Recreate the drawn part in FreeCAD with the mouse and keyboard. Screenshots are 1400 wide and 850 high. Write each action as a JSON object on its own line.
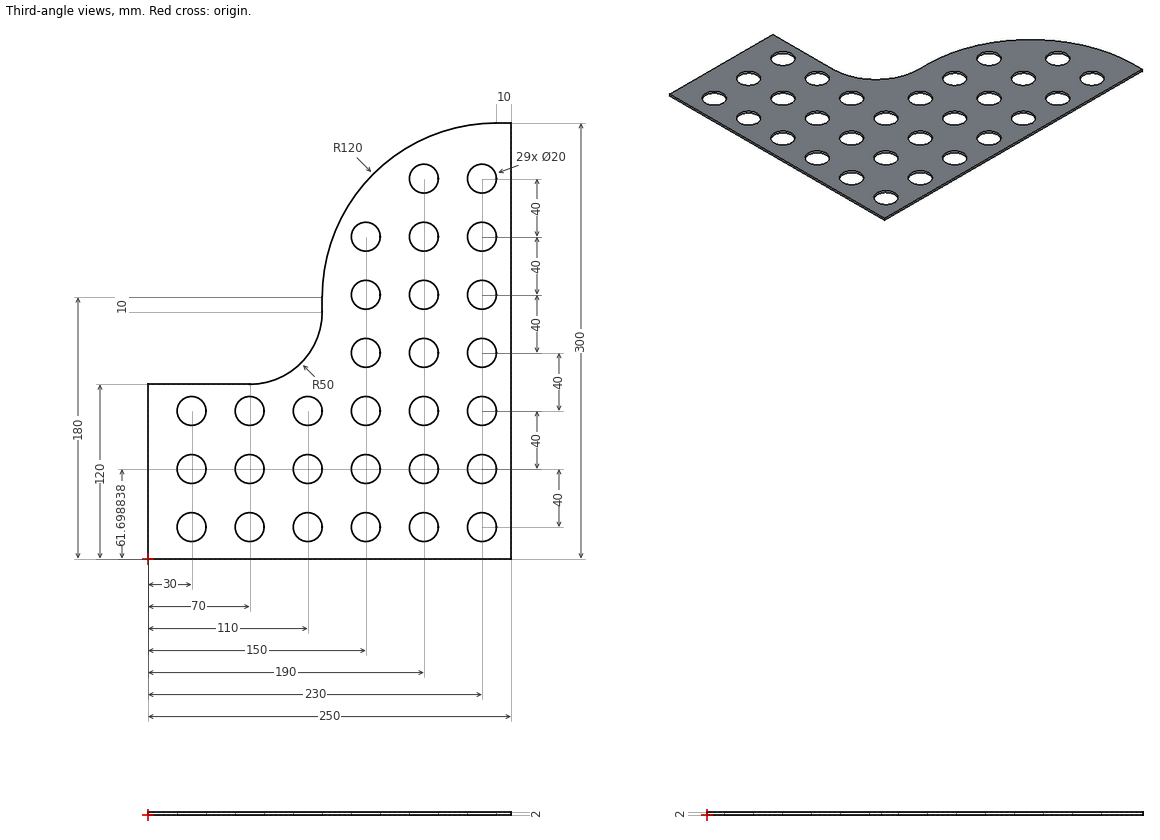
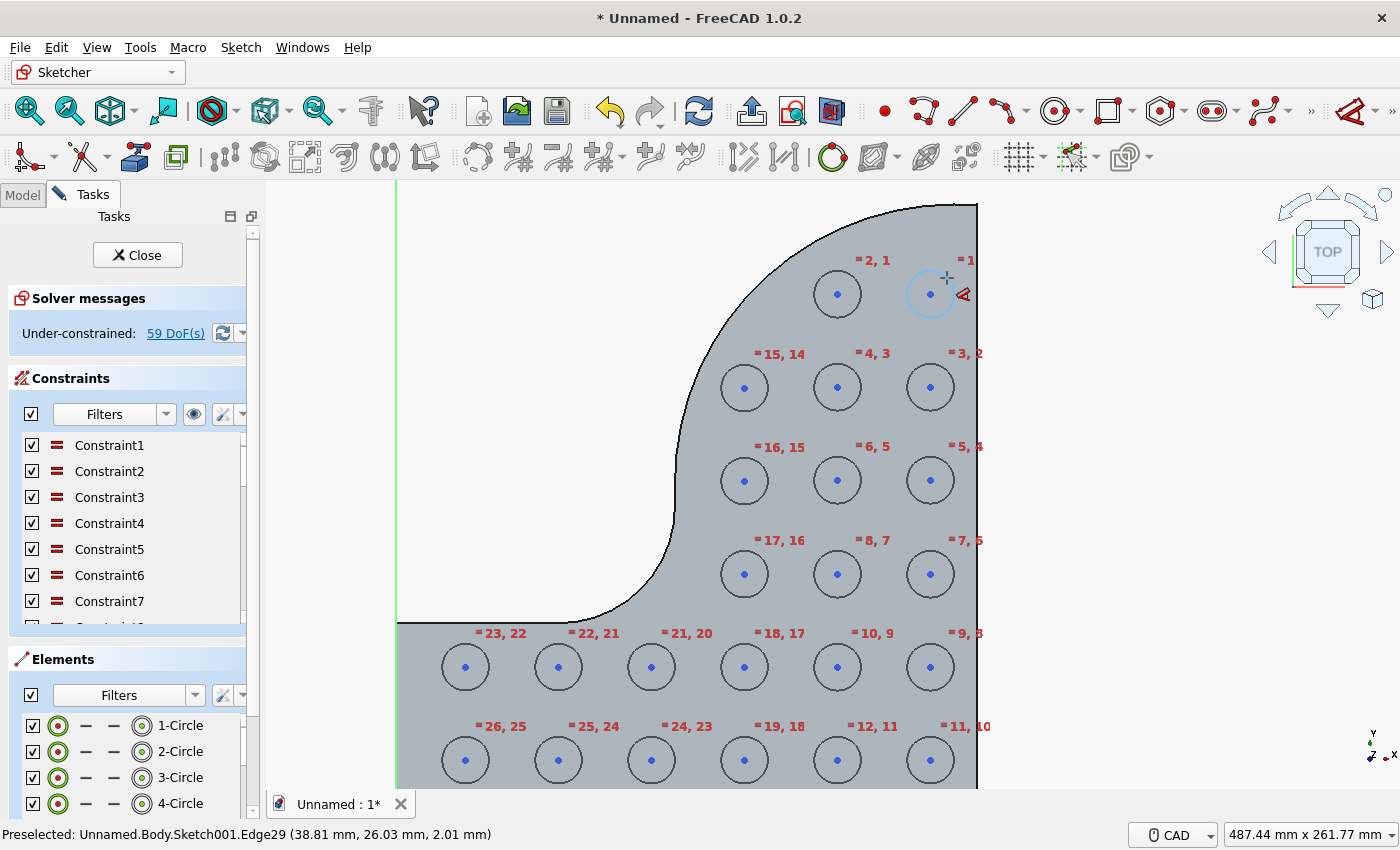
{"action": "left_click", "coordinate": [947, 278]}
{"action": "left_click", "coordinate": [970, 256]}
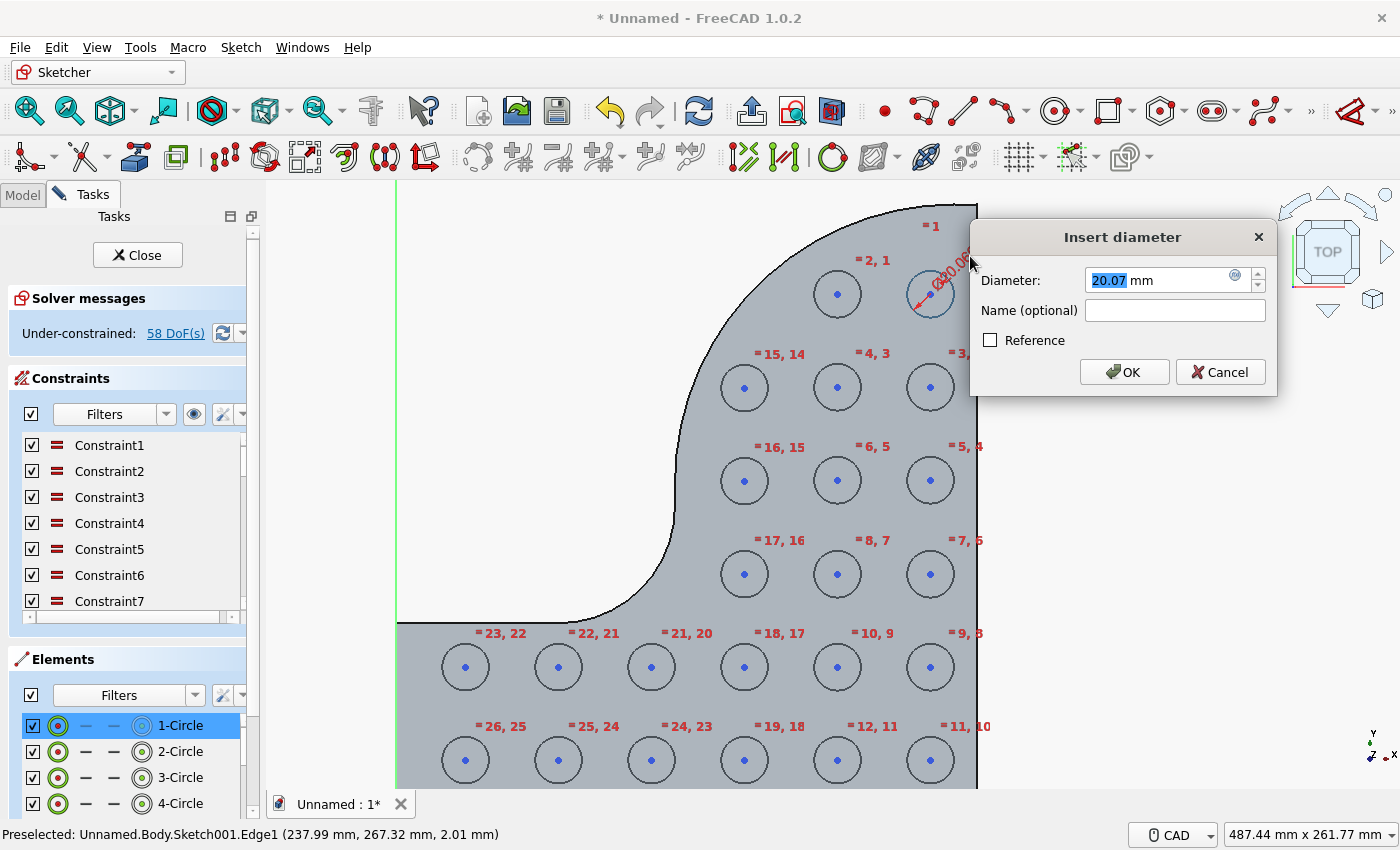
{"action": "type", "text": "20"}
{"action": "key", "text": "Return"}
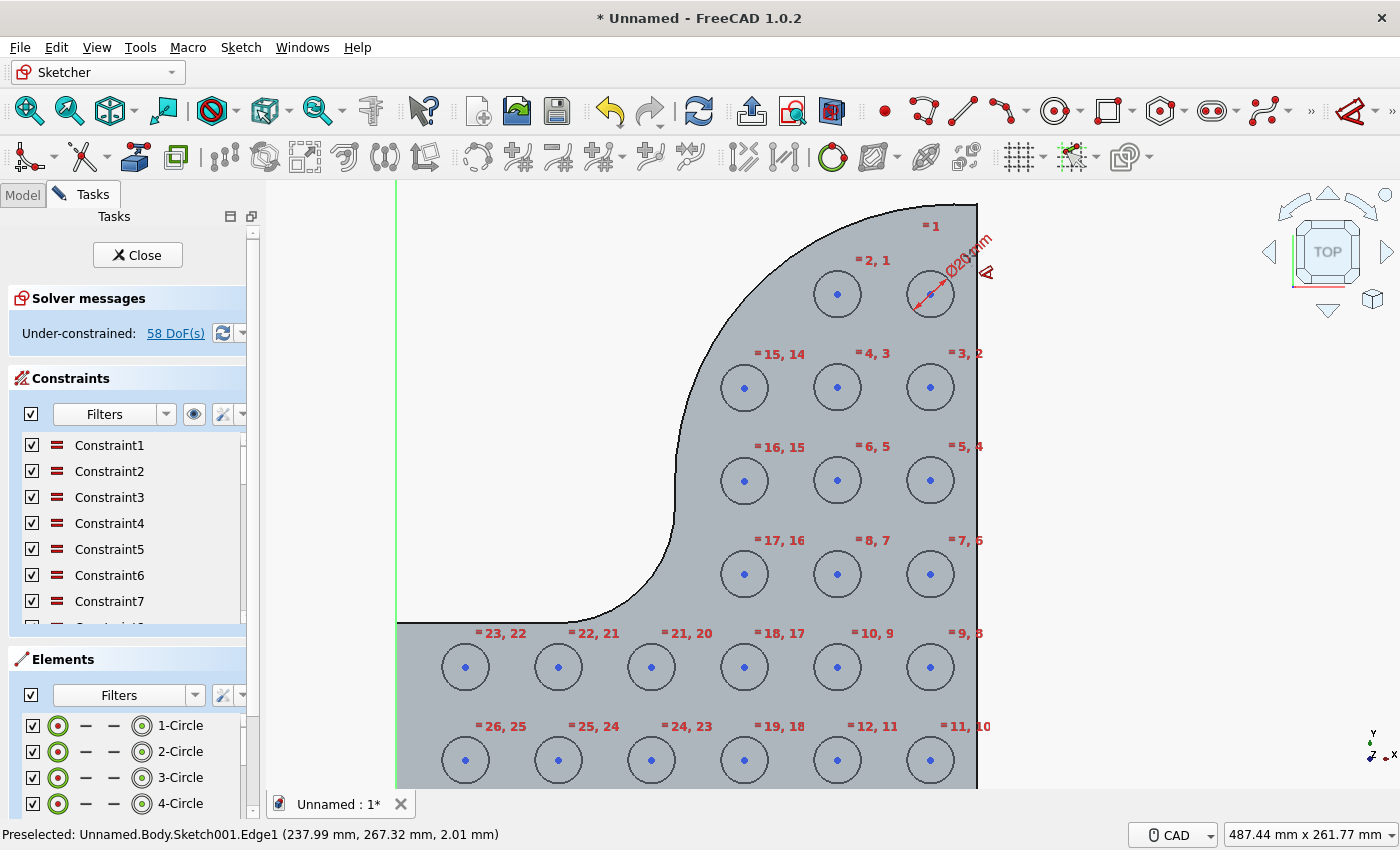
{"action": "left_click", "coordinate": [559, 667]}
{"action": "left_click", "coordinate": [440, 633]}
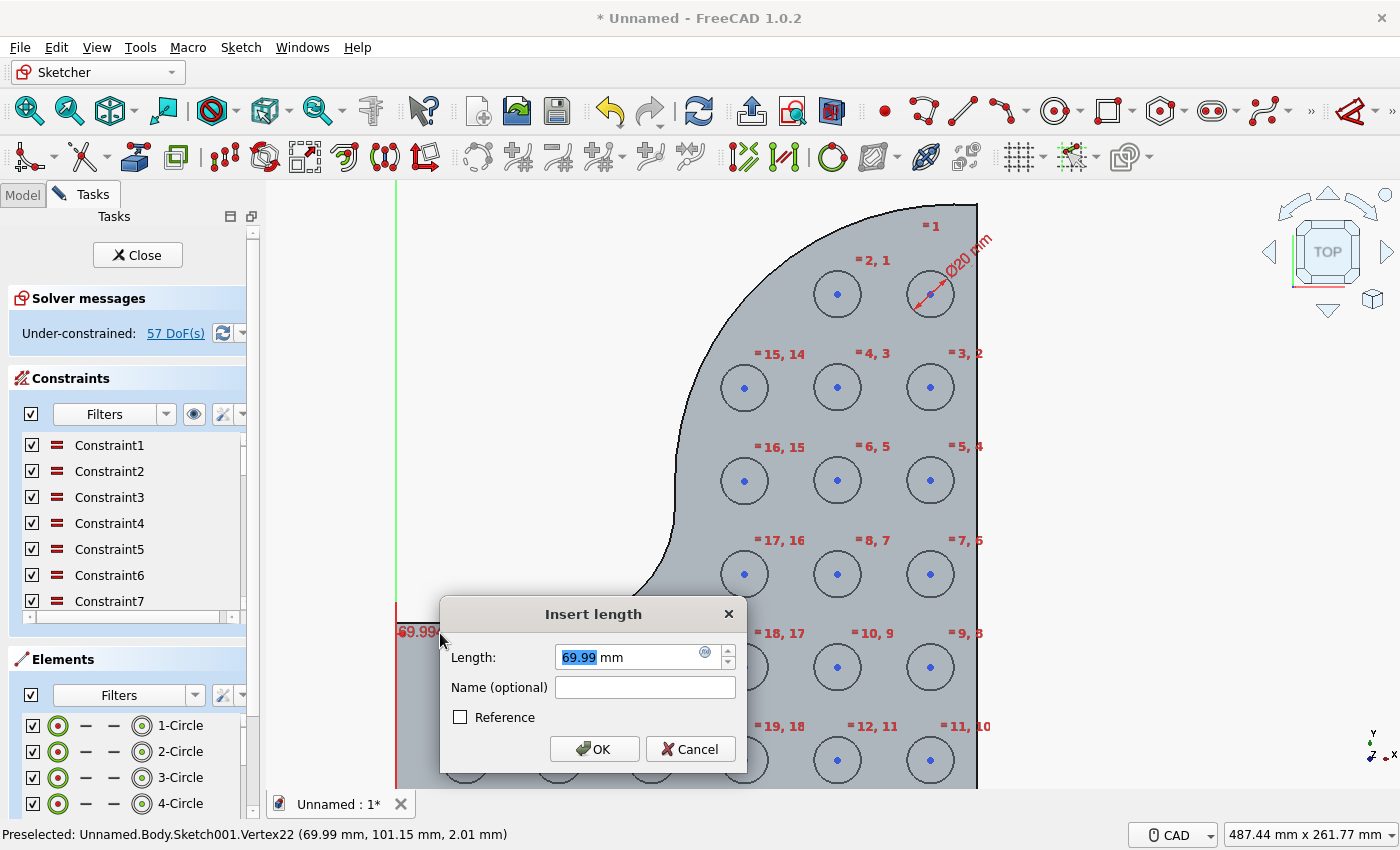
{"action": "type", "text": "70"}
{"action": "key", "text": "Return"}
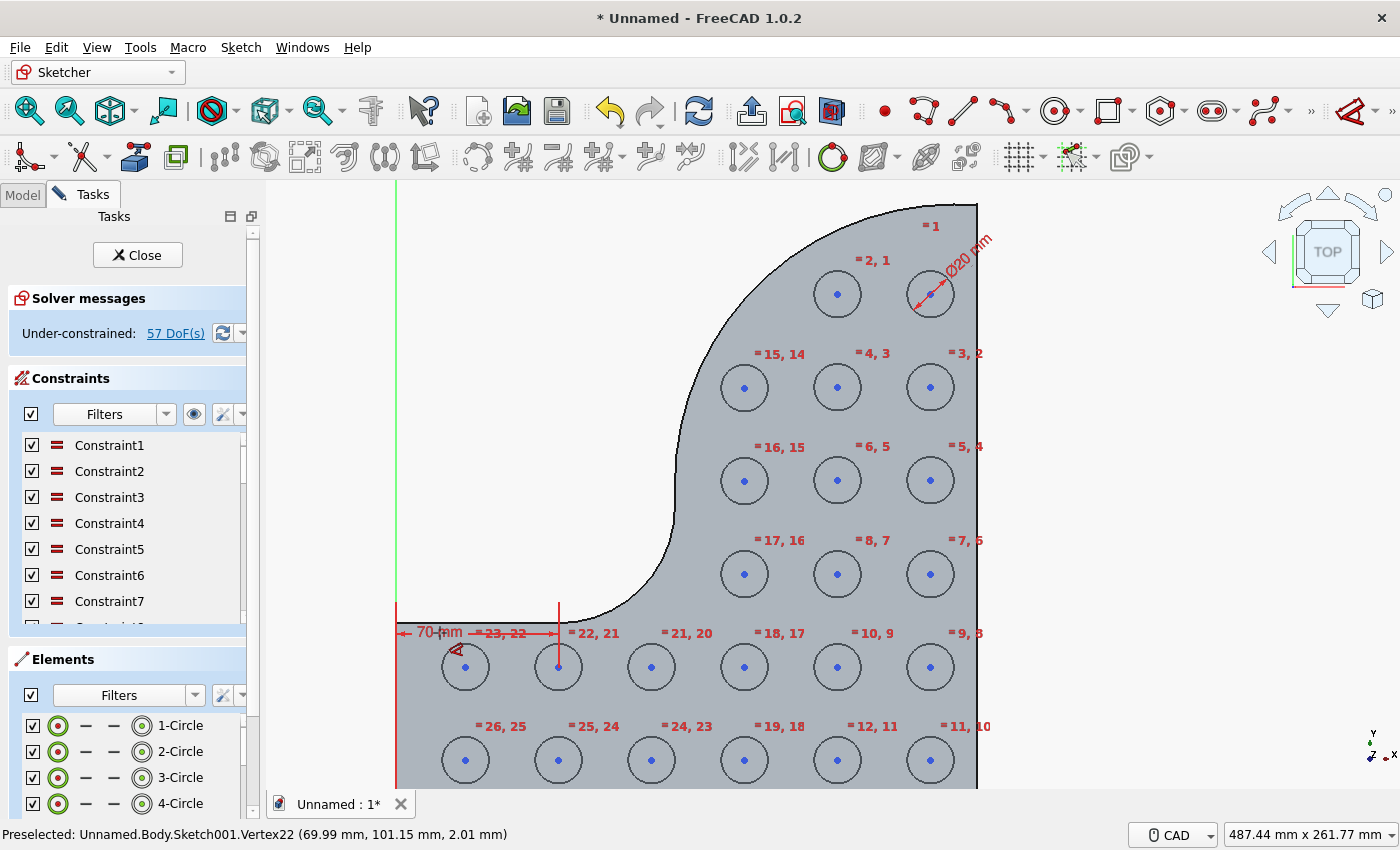
{"action": "left_click", "coordinate": [466, 667]}
{"action": "left_click", "coordinate": [431, 609]}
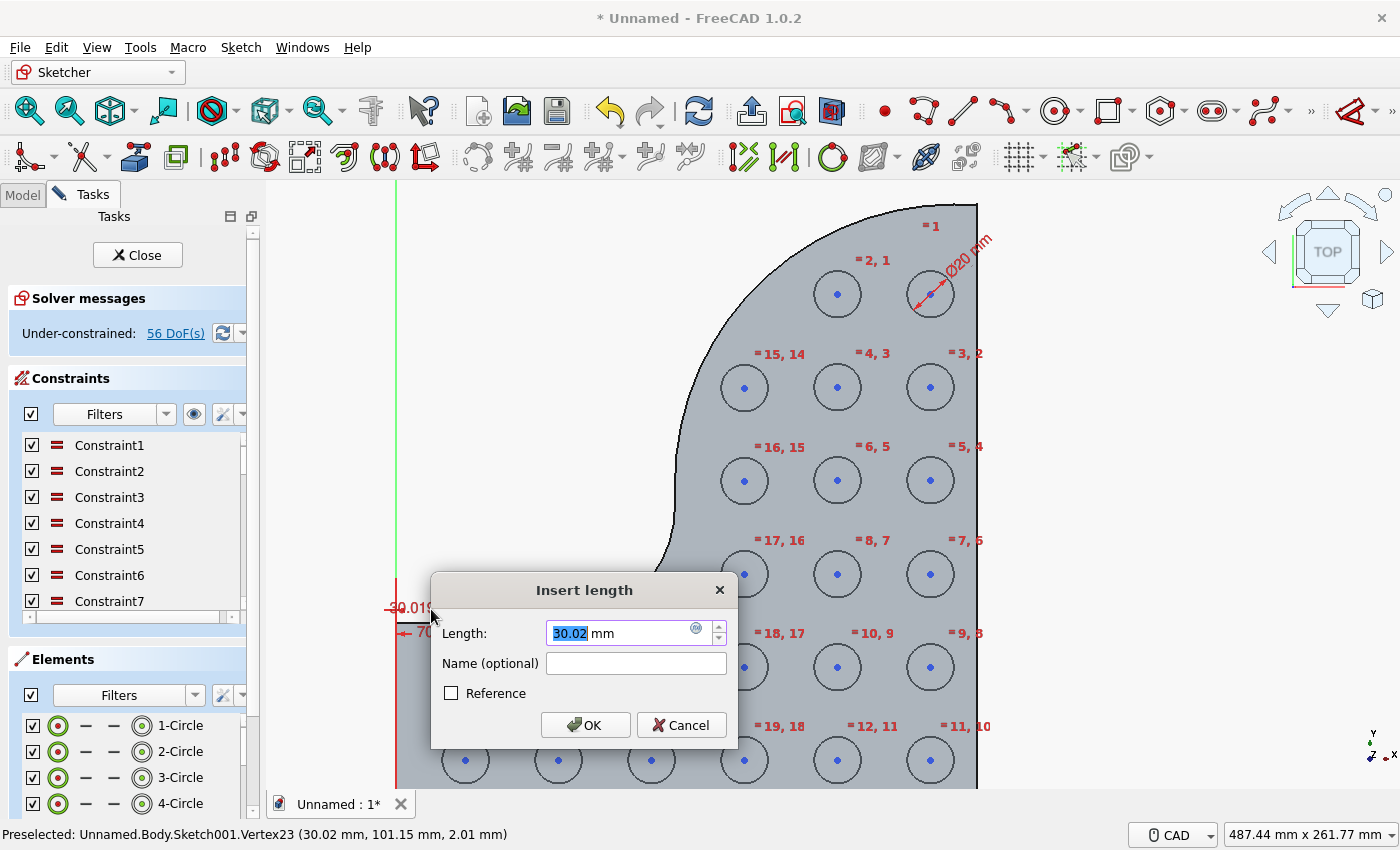
{"action": "type", "text": "30"}
{"action": "key", "text": "Return"}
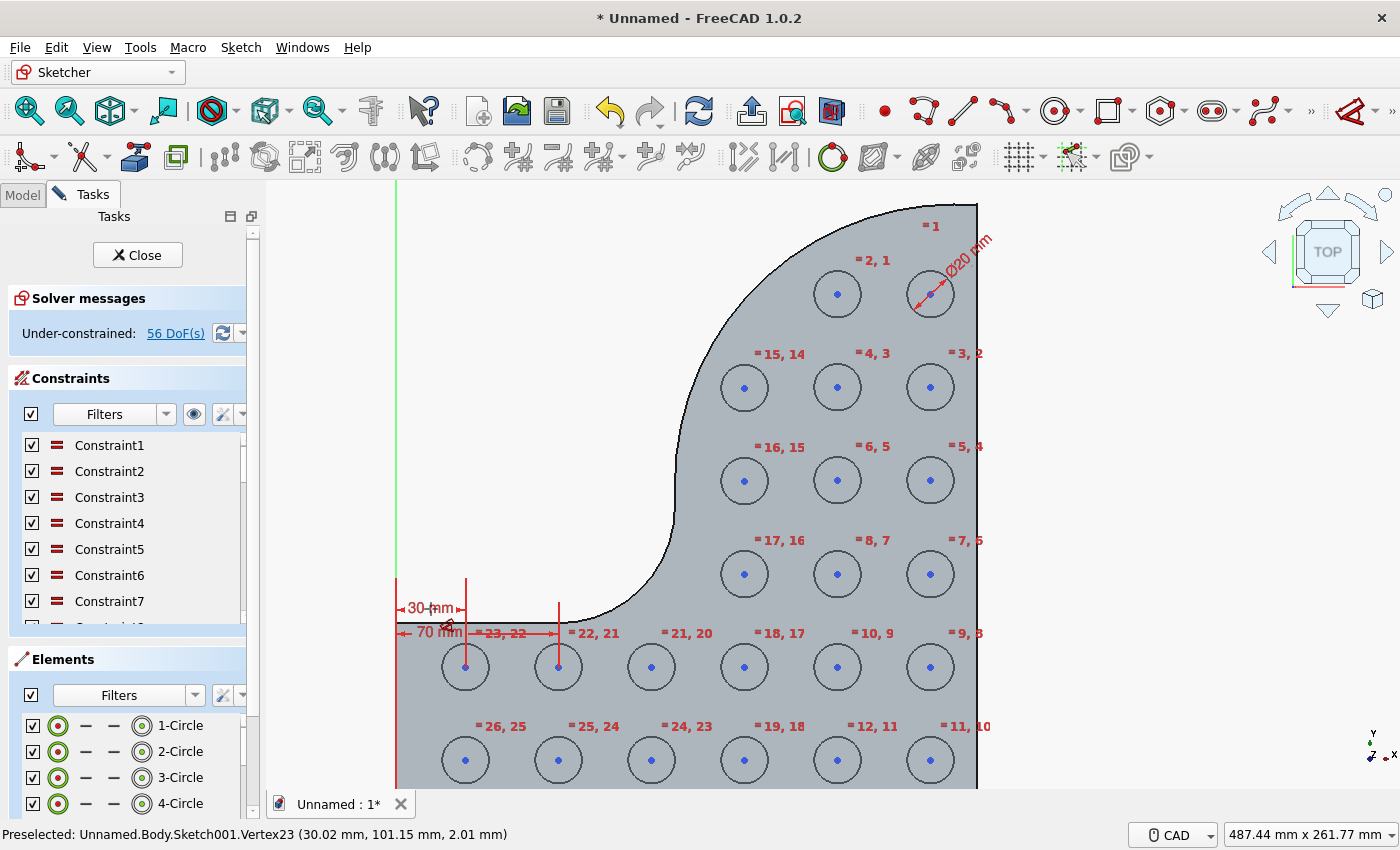
{"action": "left_click", "coordinate": [559, 760]}
{"action": "left_click", "coordinate": [440, 726]}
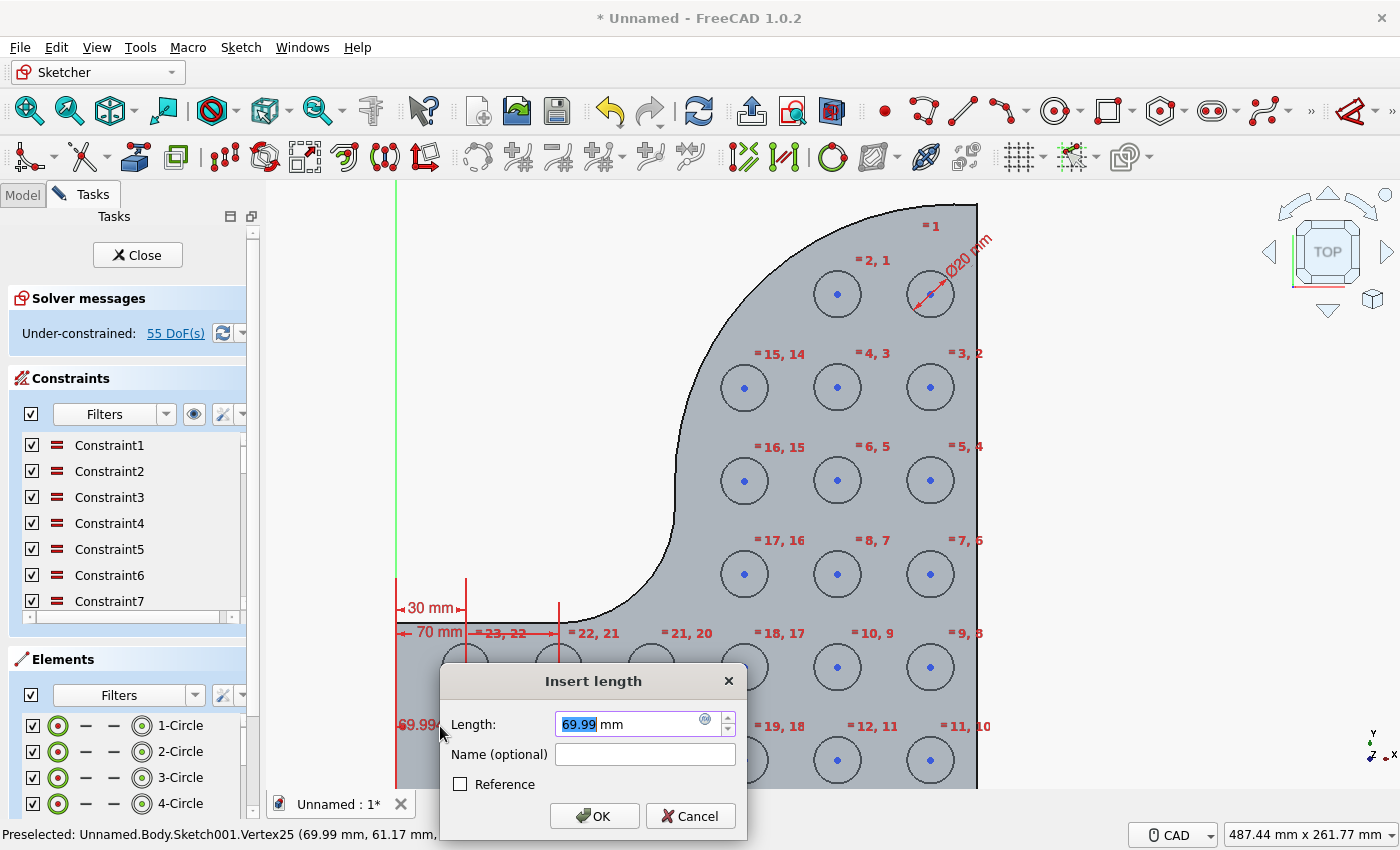
{"action": "type", "text": "70"}
{"action": "key", "text": "Return"}